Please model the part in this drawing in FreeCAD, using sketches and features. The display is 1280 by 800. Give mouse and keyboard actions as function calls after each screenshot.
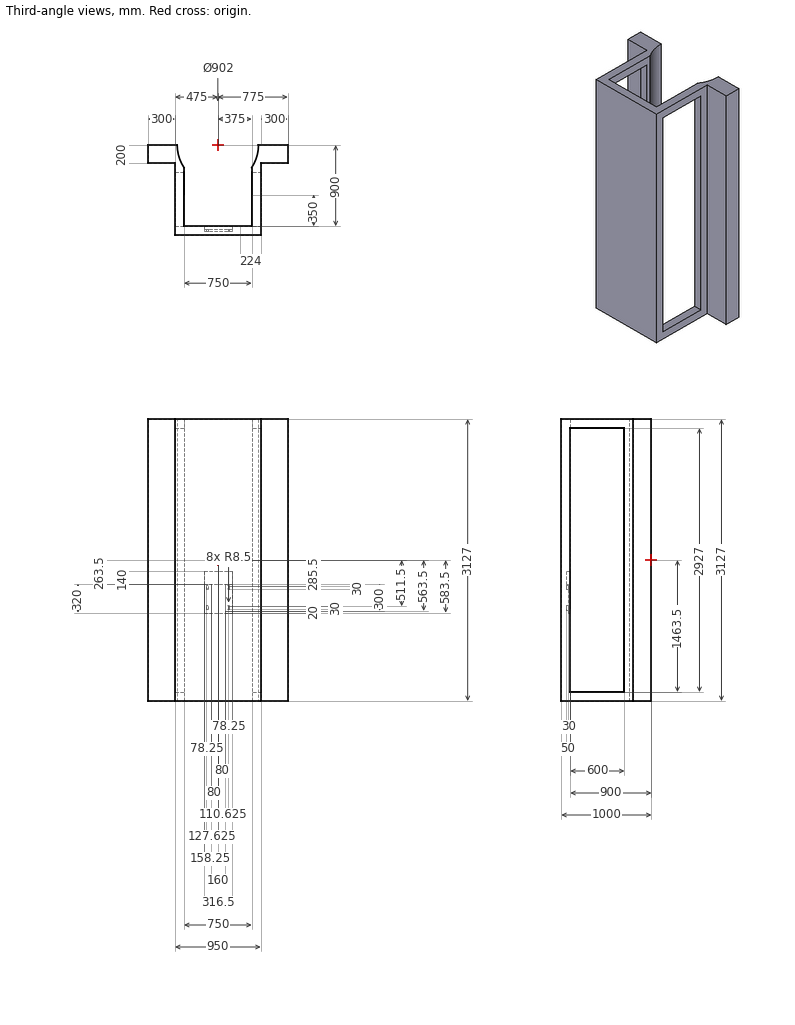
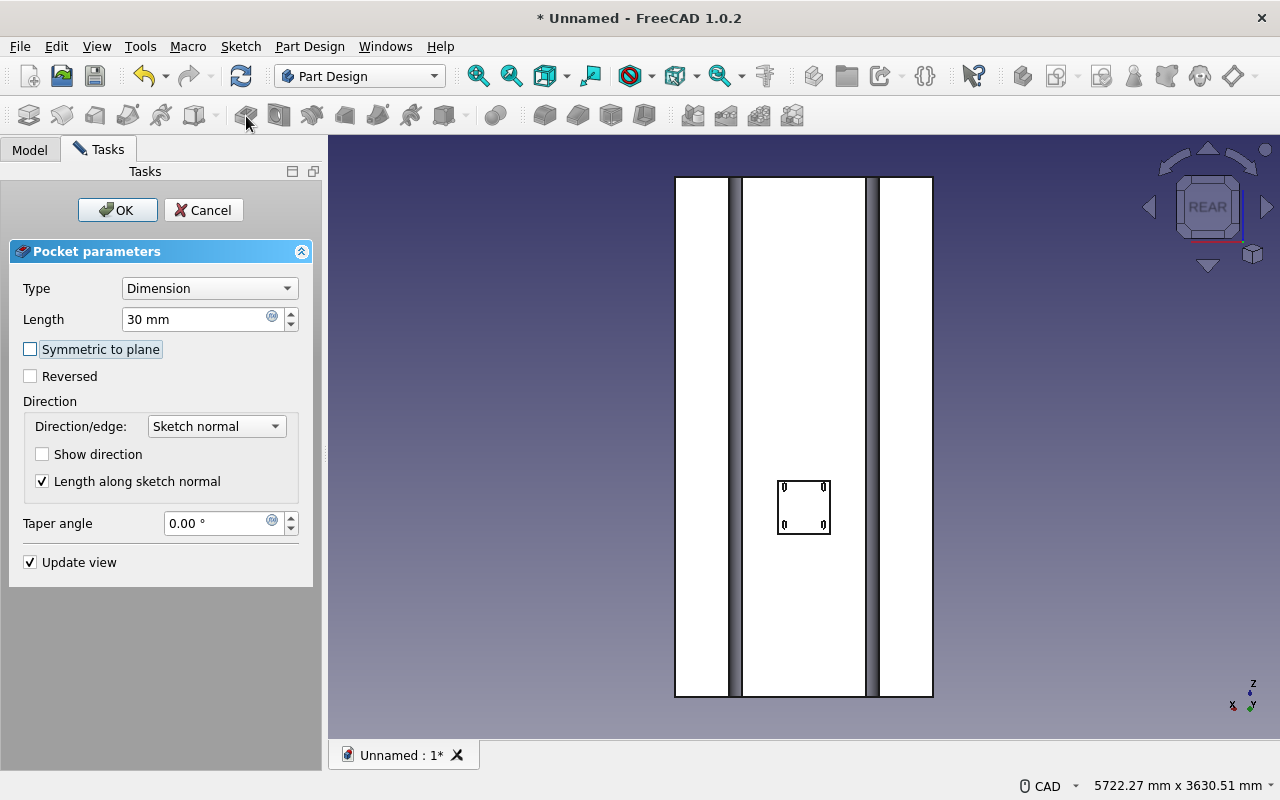
click(118, 210)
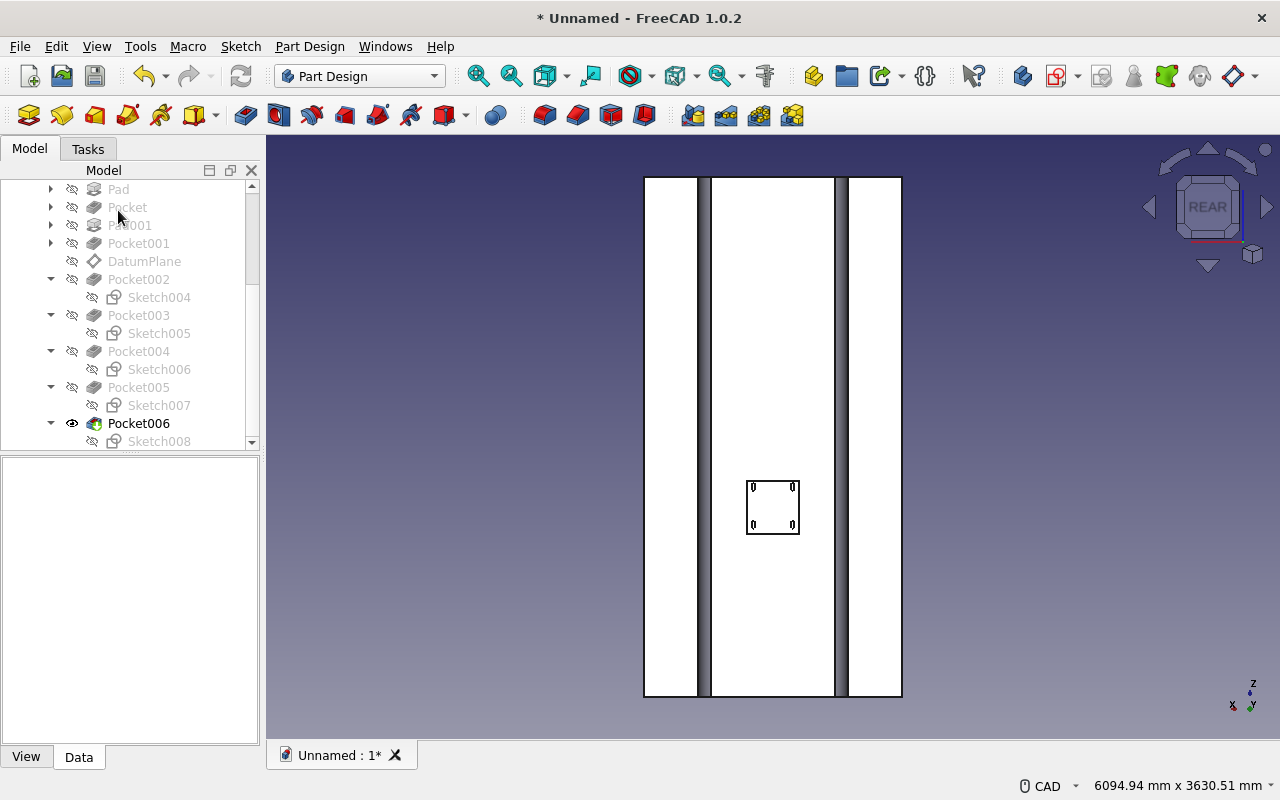
key(0)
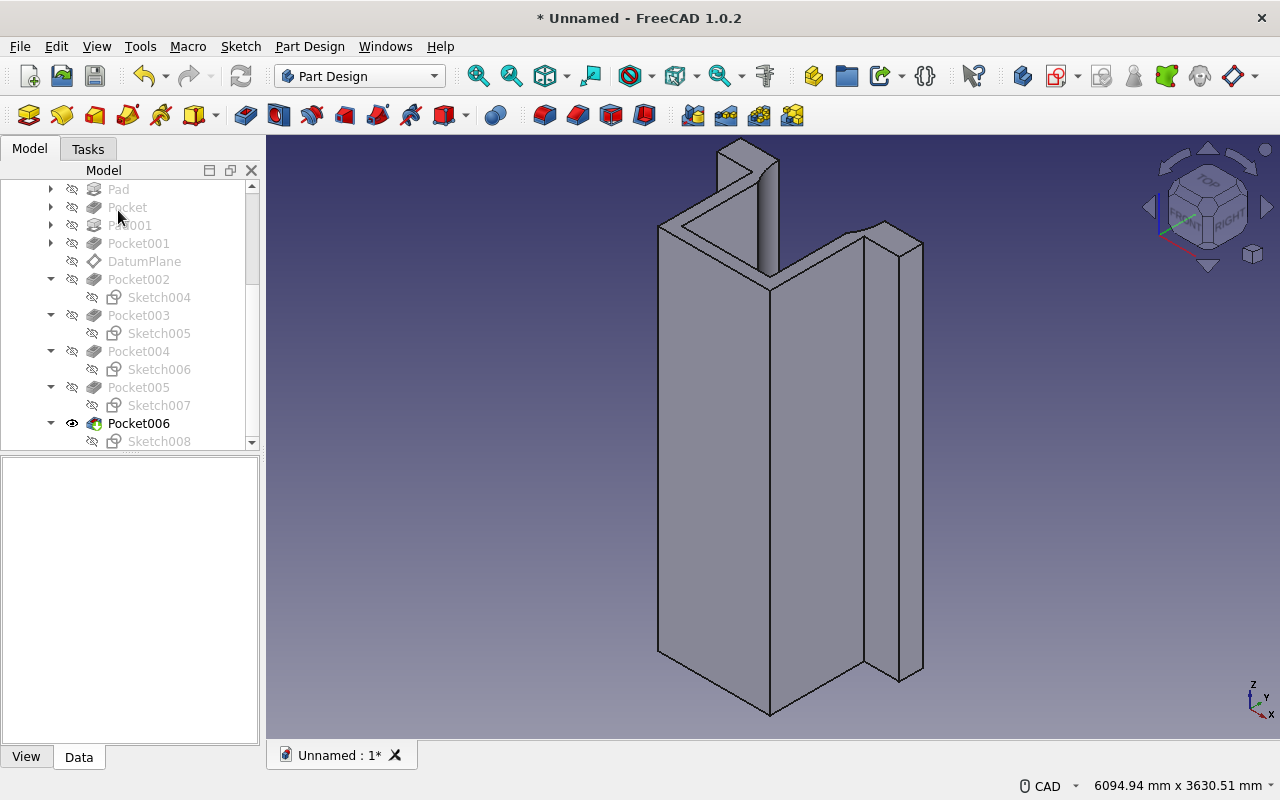
click(817, 536)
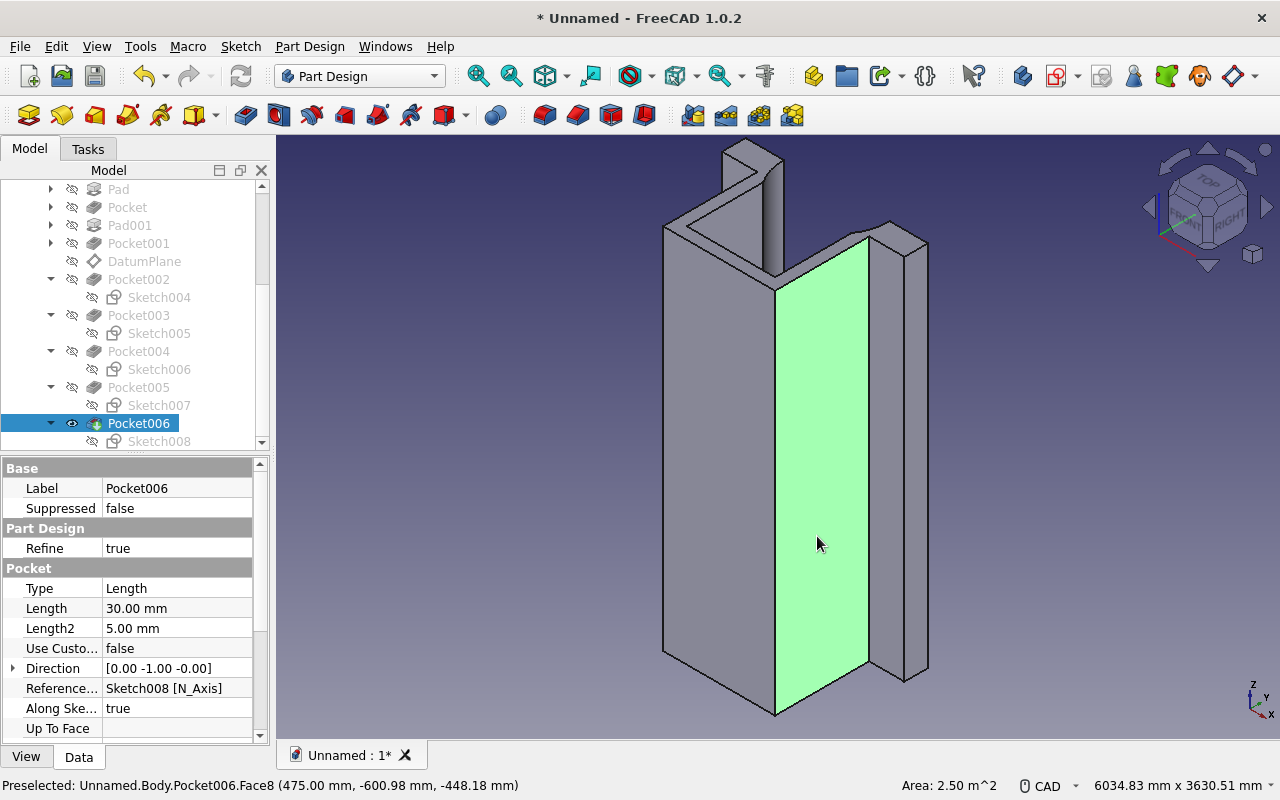
click(1056, 76)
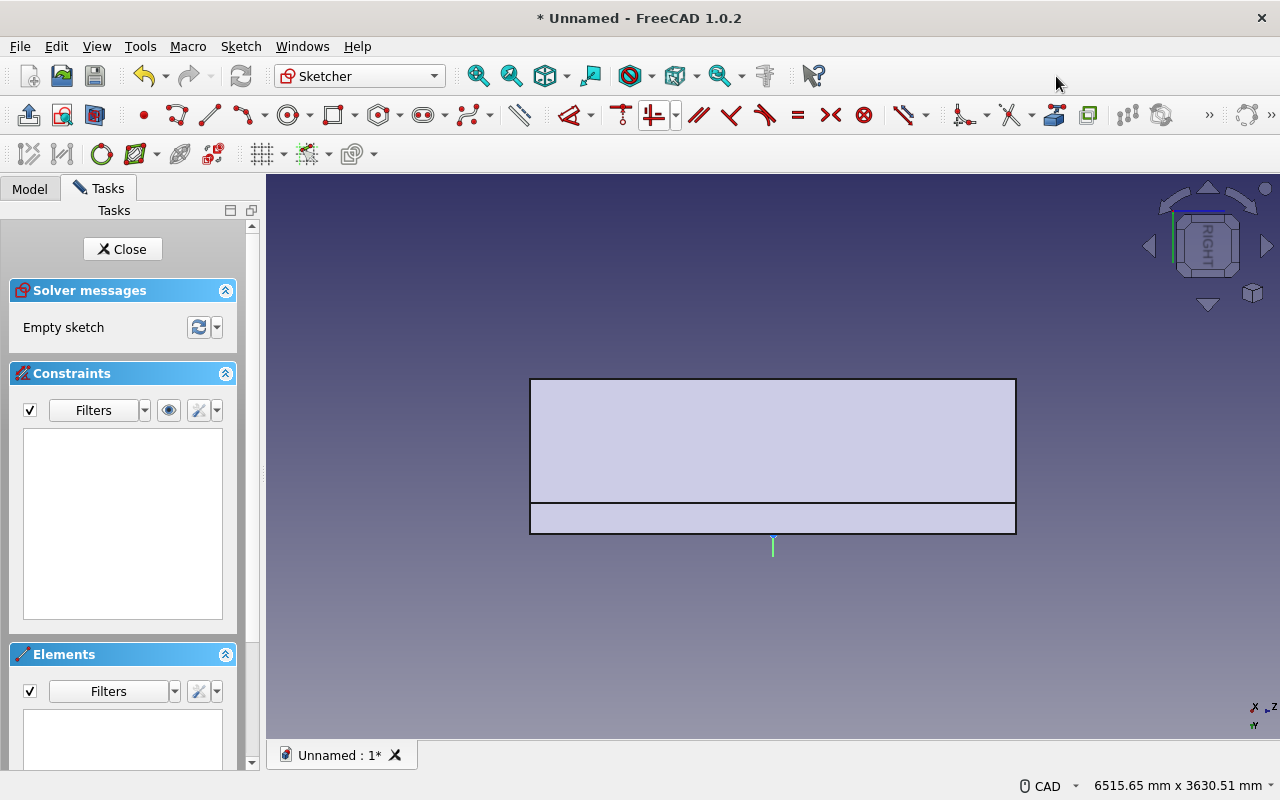
click(332, 116)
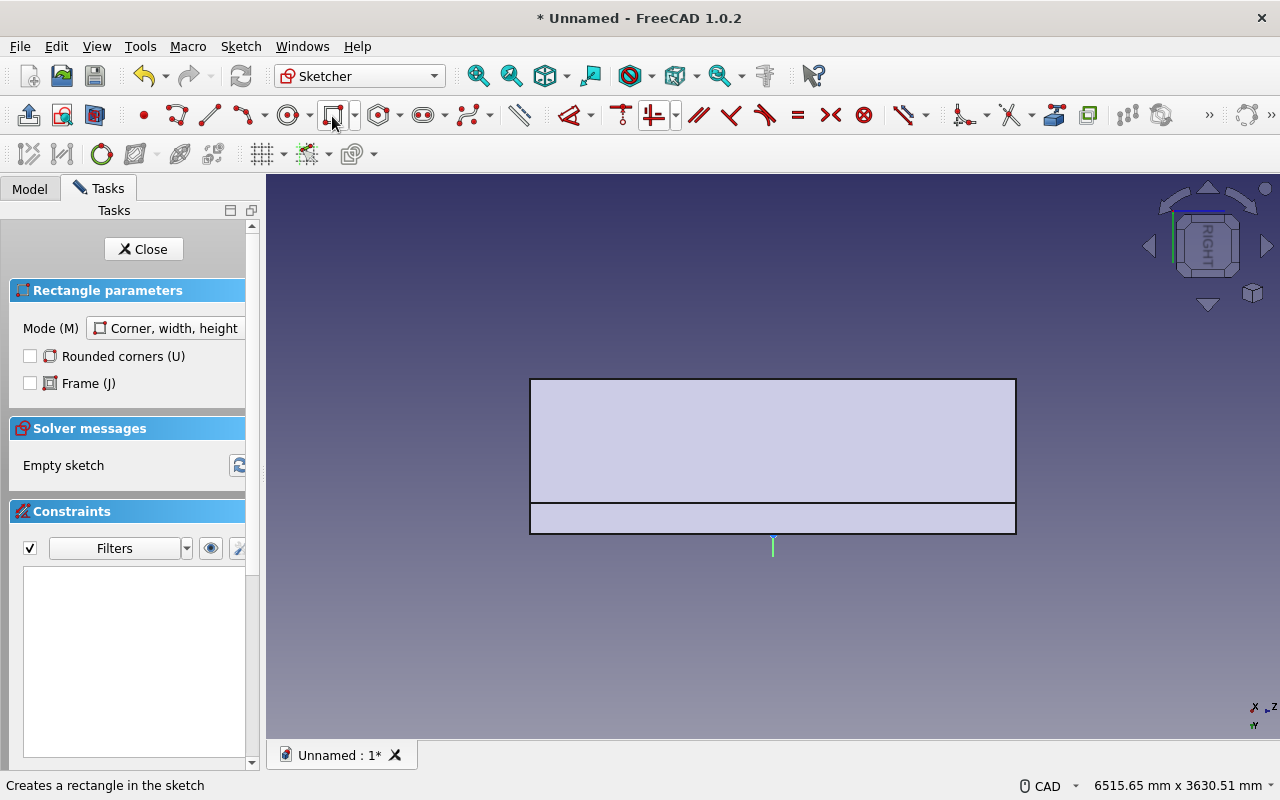
click(545, 394)
click(1001, 488)
key(Escape)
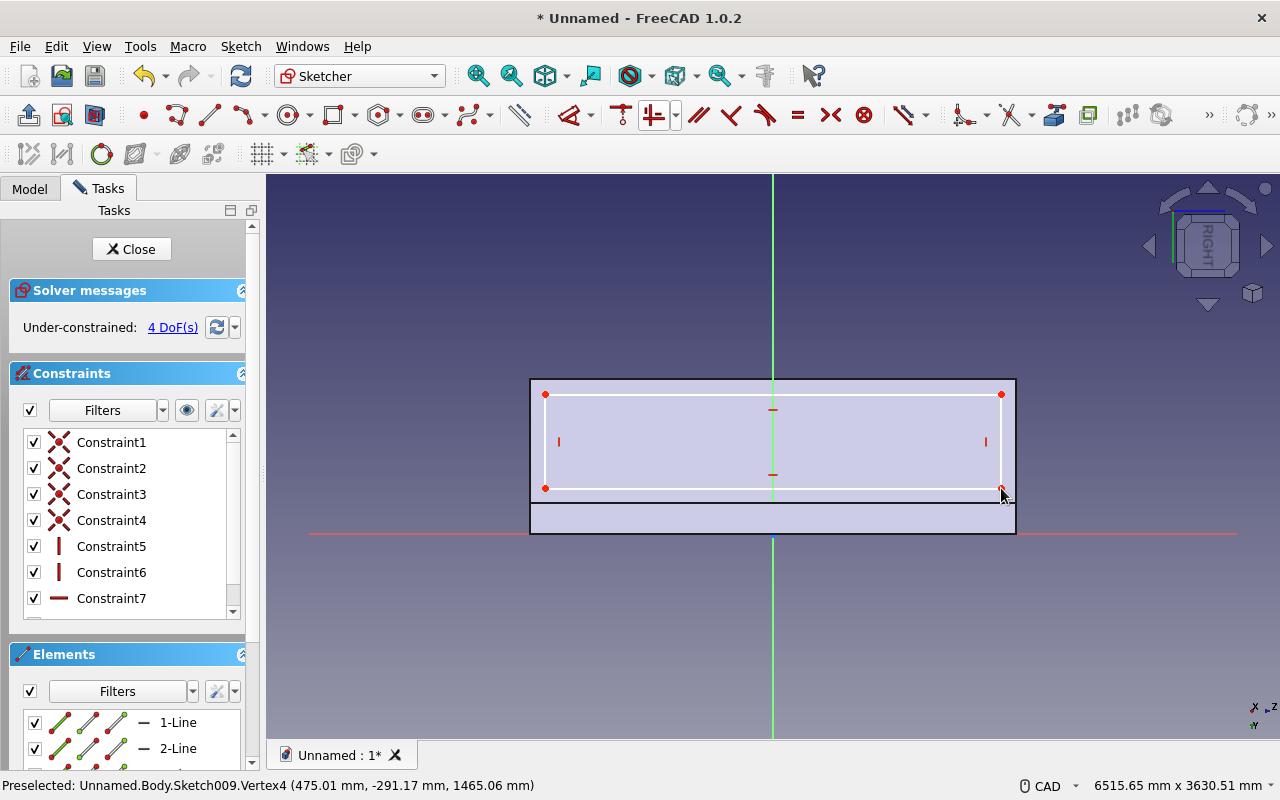
click(568, 116)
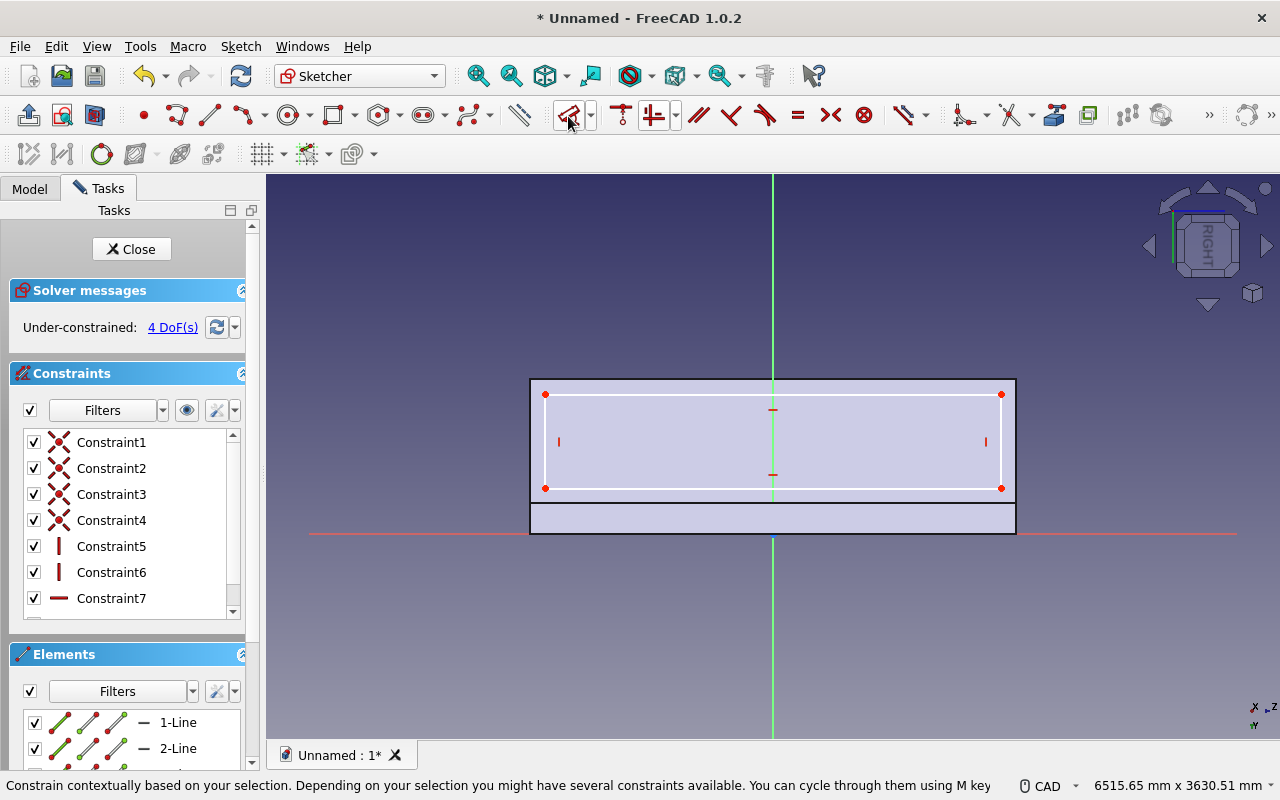
click(545, 423)
click(511, 442)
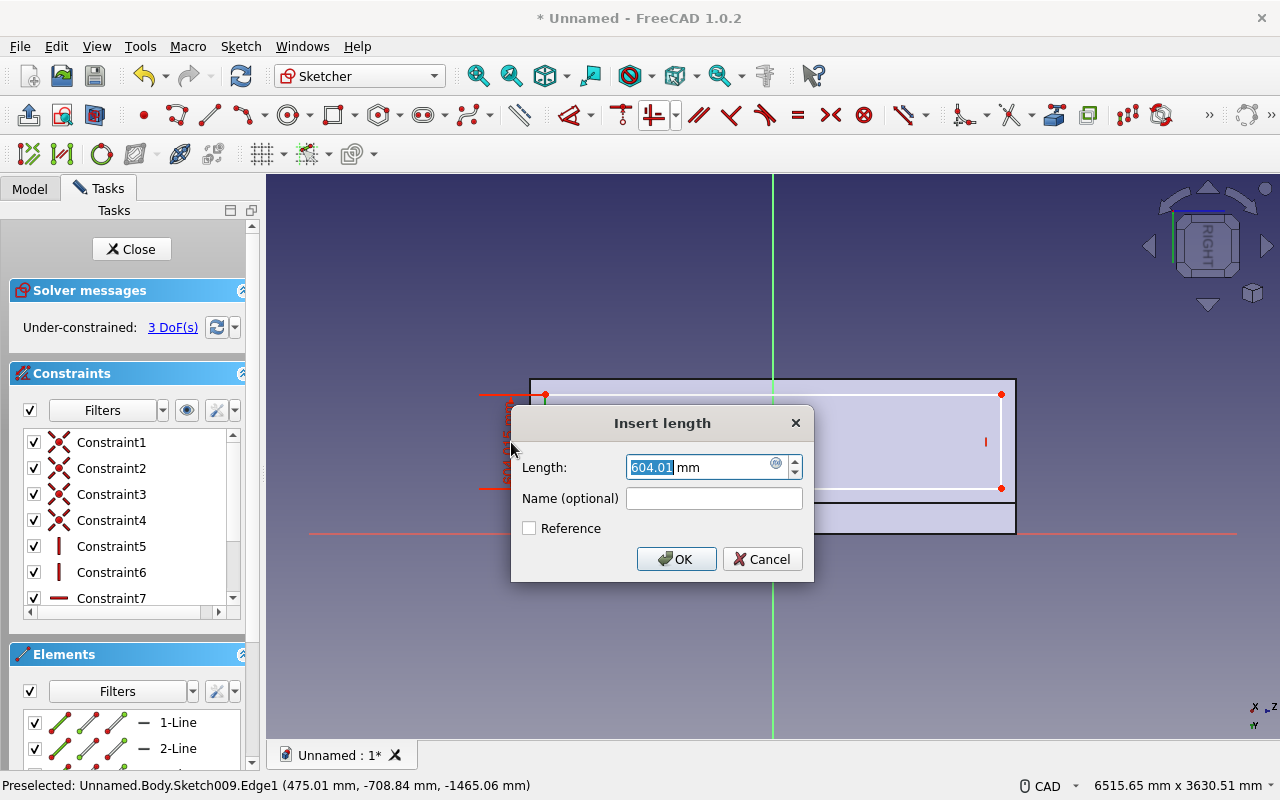
text(600)
key(Return)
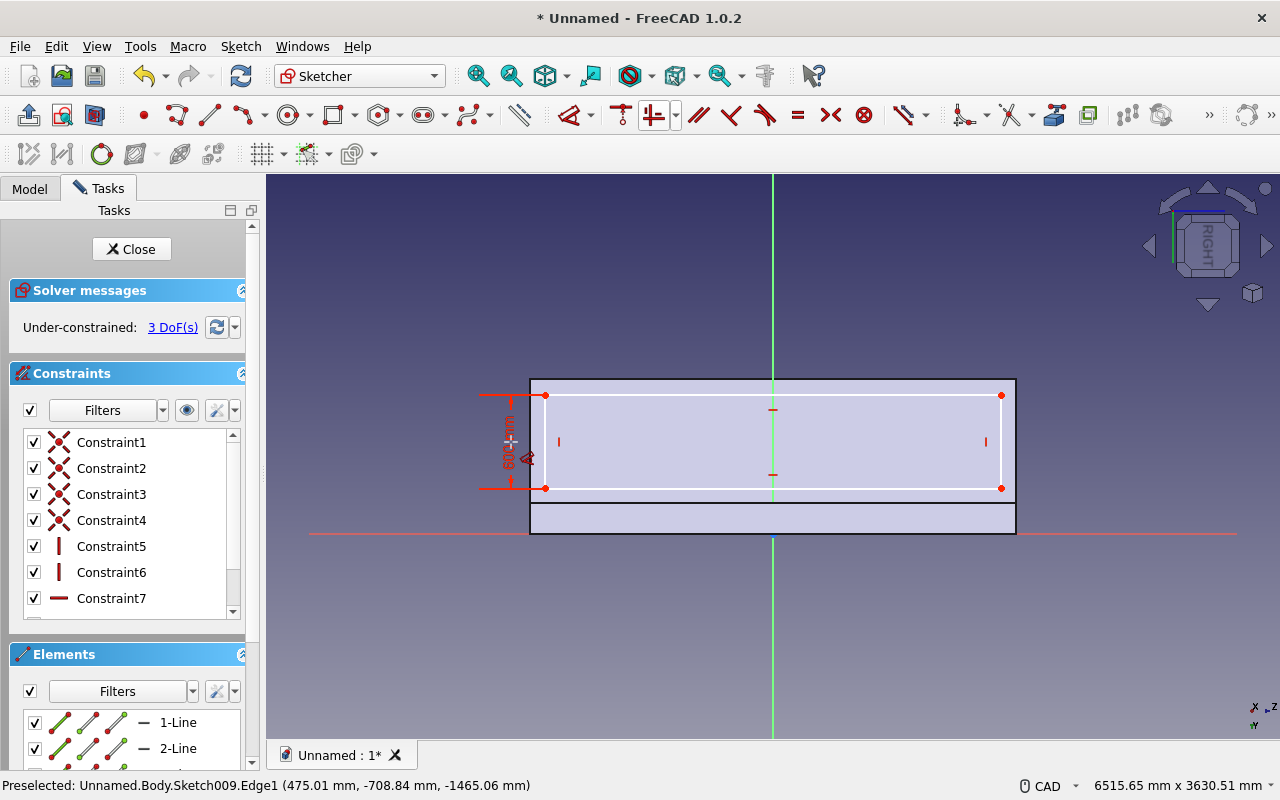
click(682, 489)
click(668, 455)